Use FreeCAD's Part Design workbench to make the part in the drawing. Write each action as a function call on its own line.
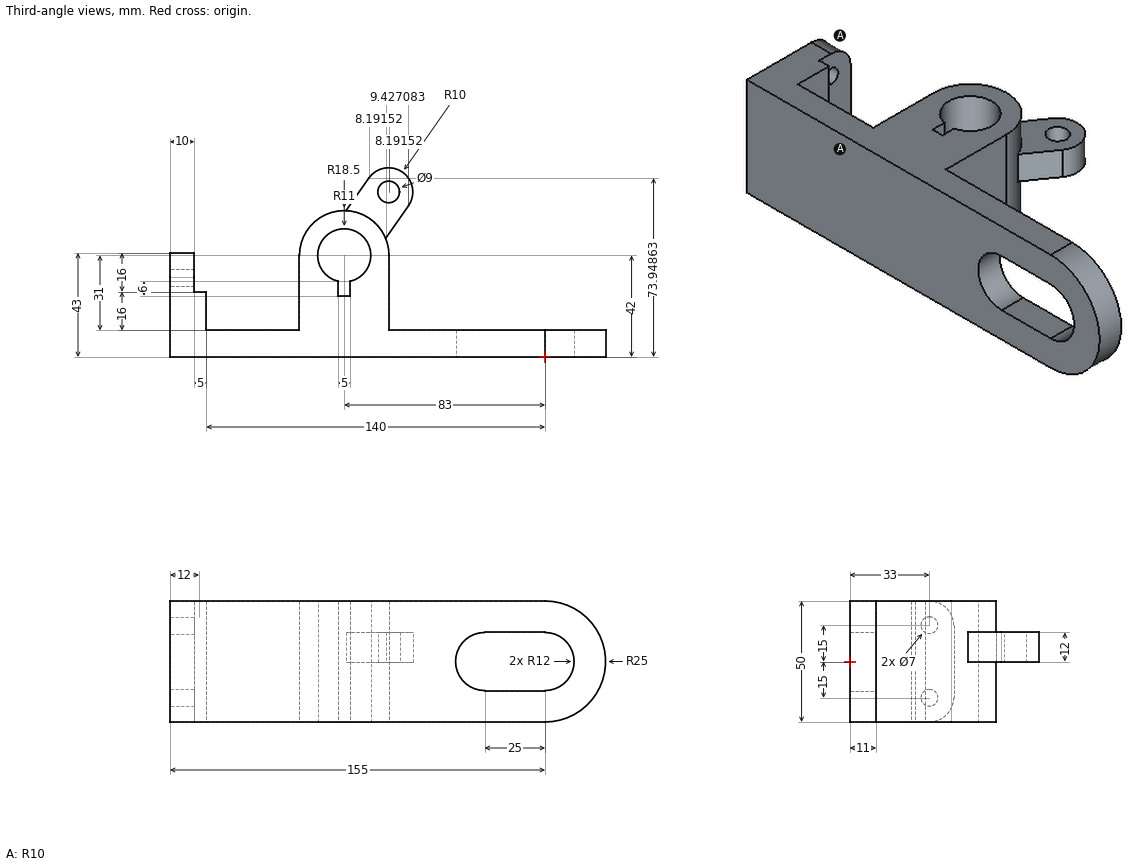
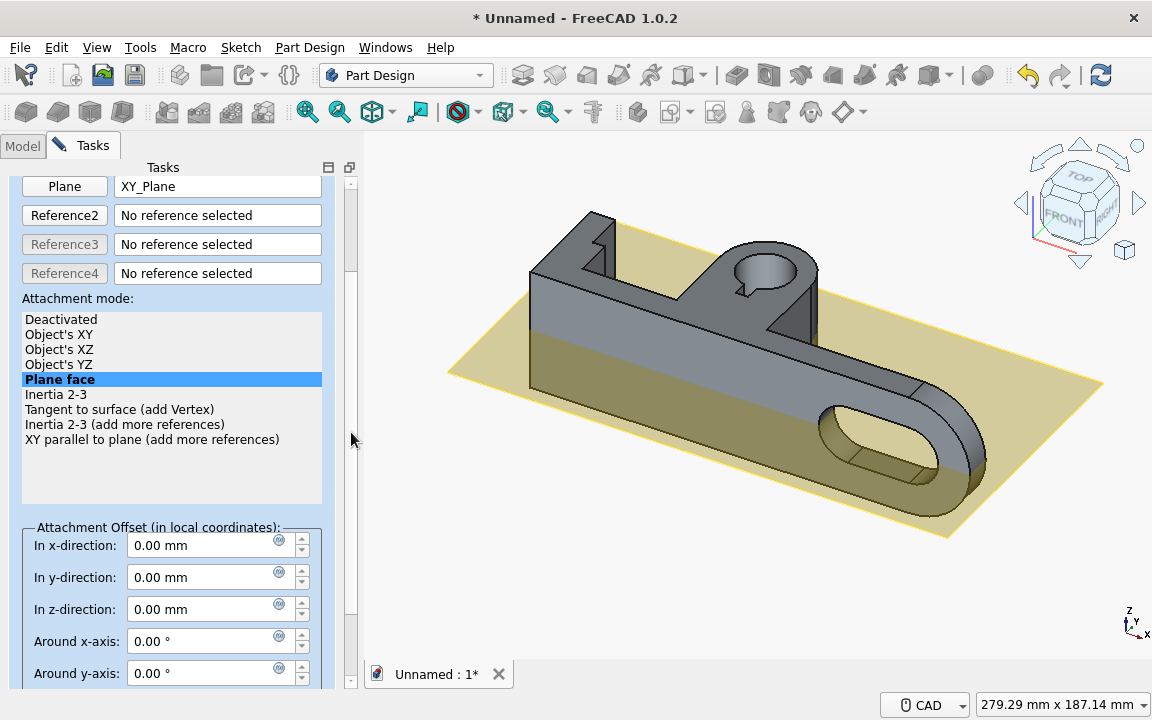
triple_click(210, 609)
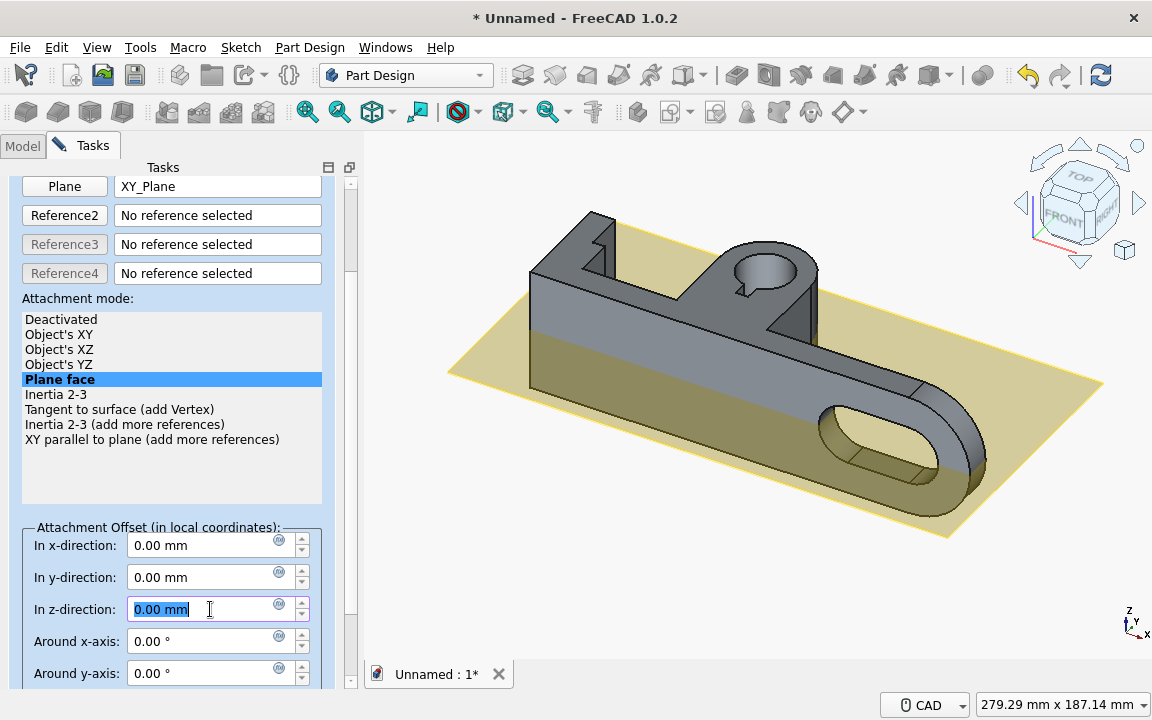
text(12)
key(Tab)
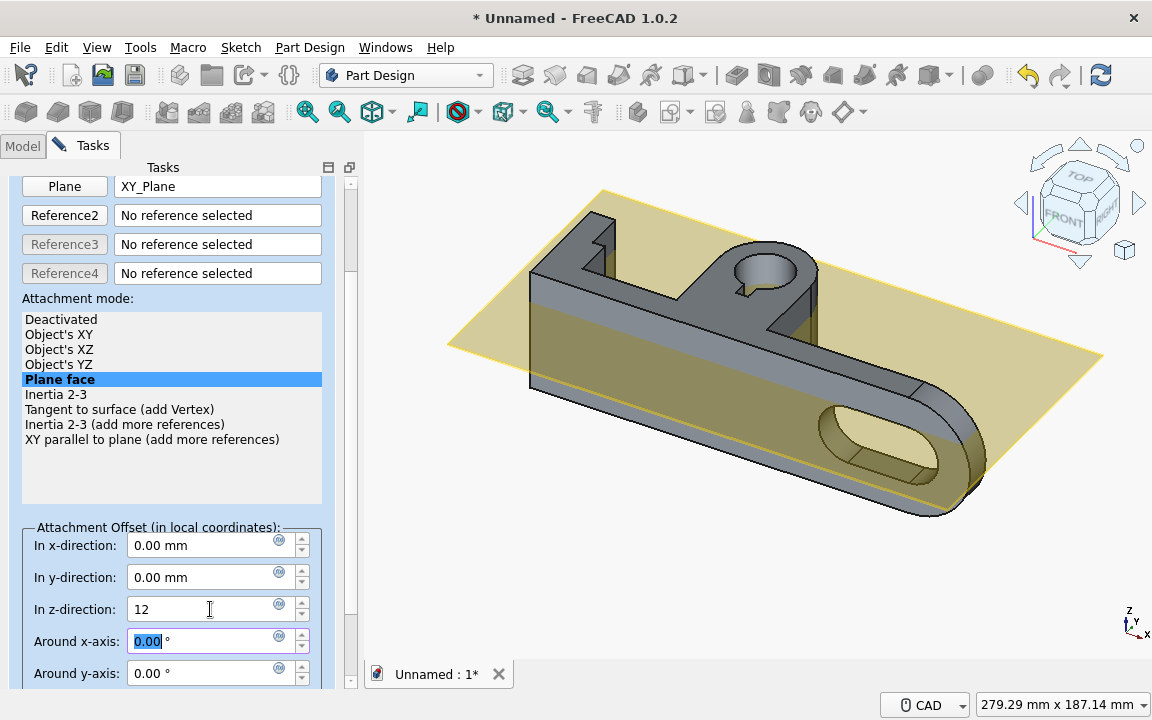
scroll(351, 432, up, 3)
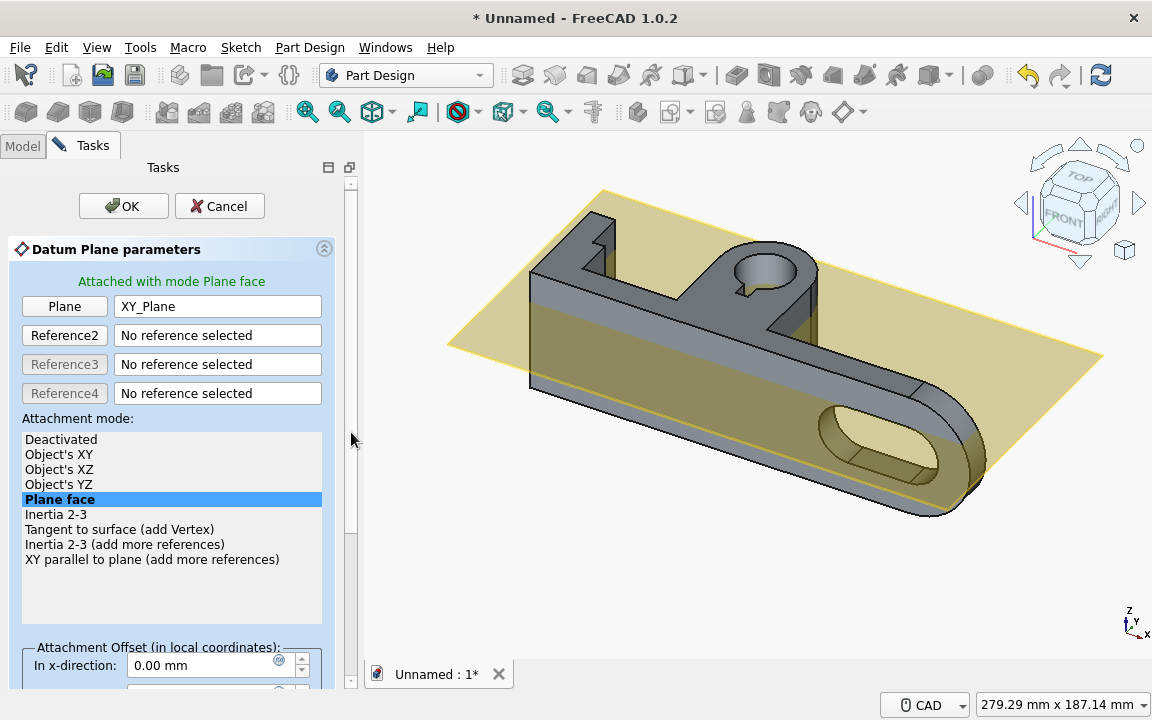
click(124, 206)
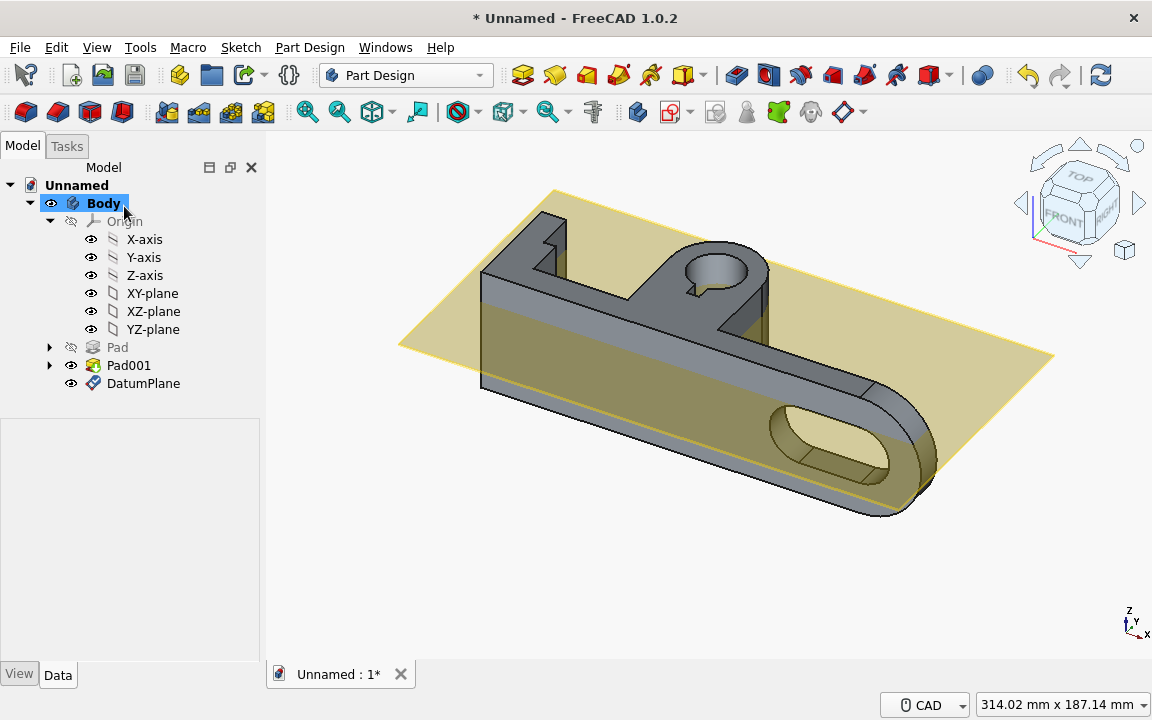
click(116, 383)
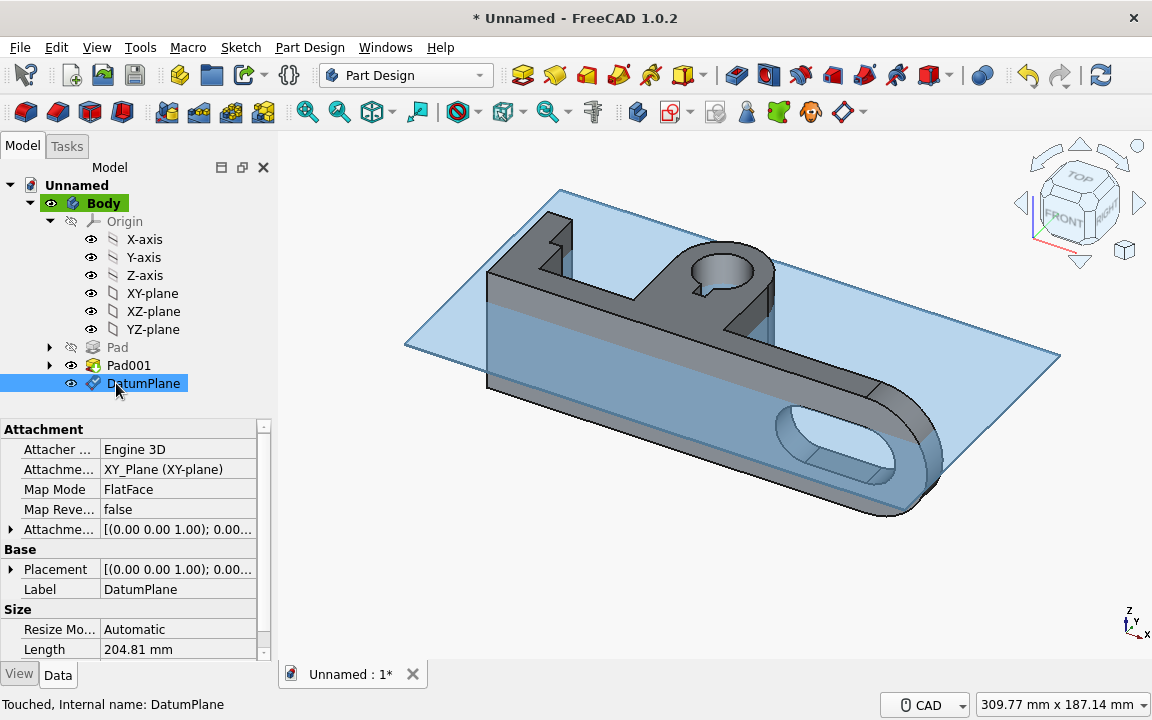
click(670, 112)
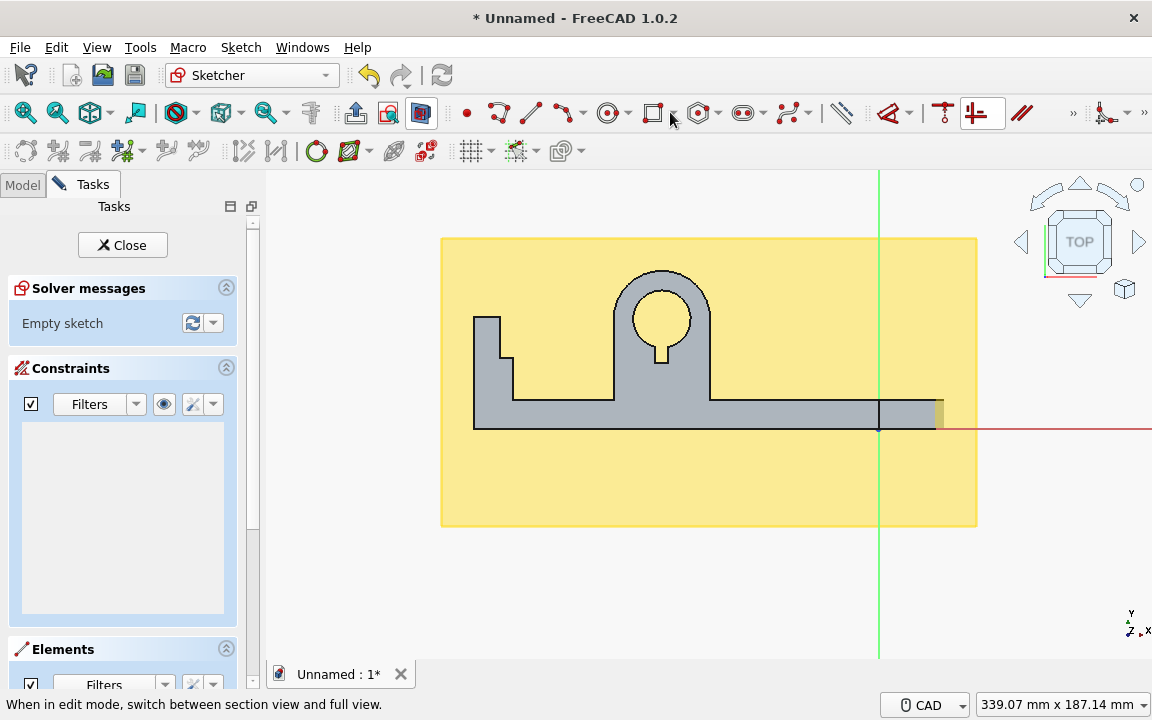
click(422, 114)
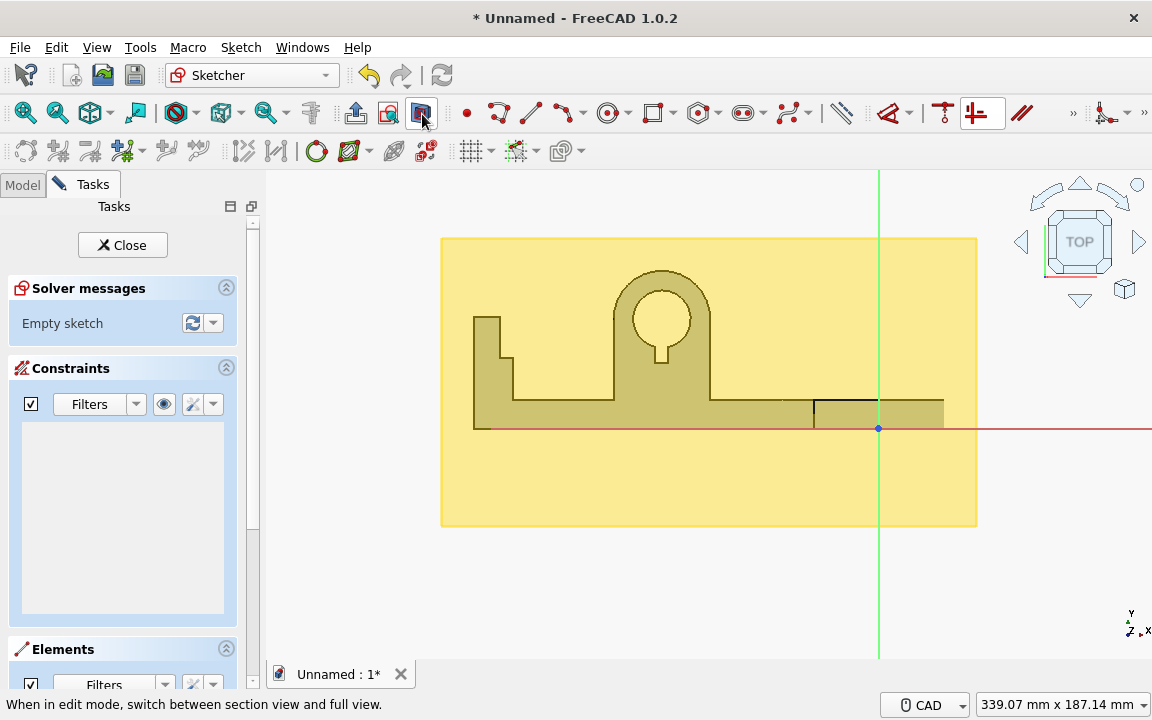
scroll(716, 216, up, 7)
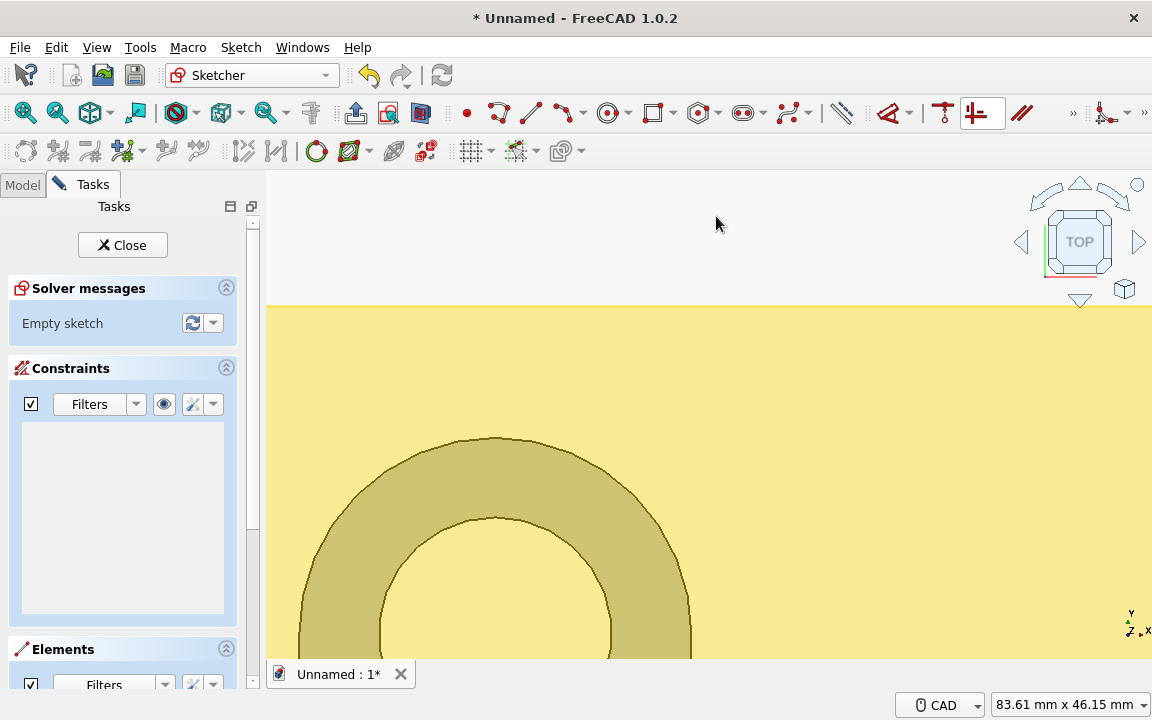
click(532, 114)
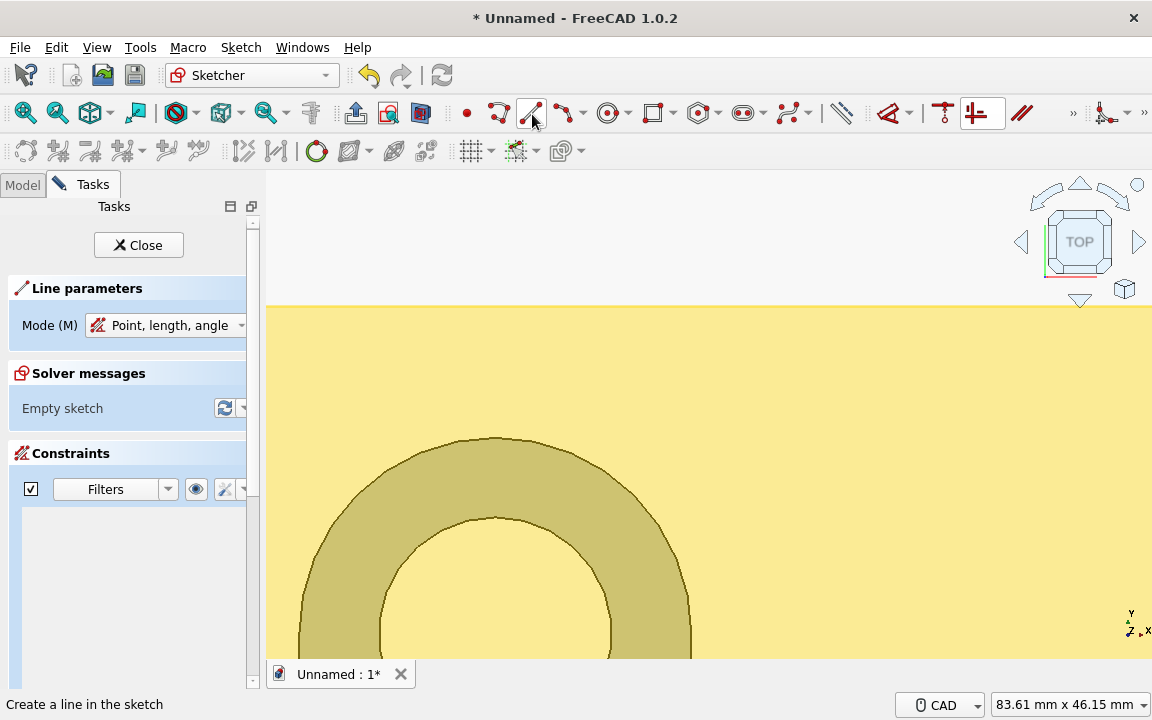
click(677, 560)
click(777, 417)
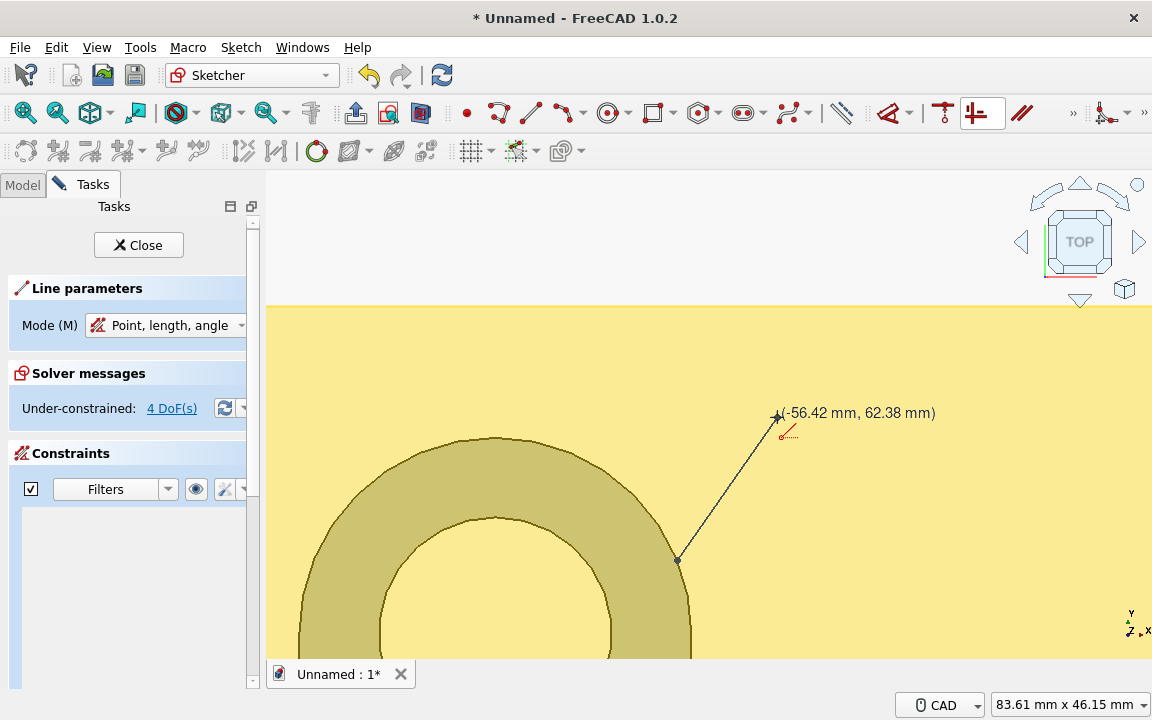
click(603, 295)
click(503, 438)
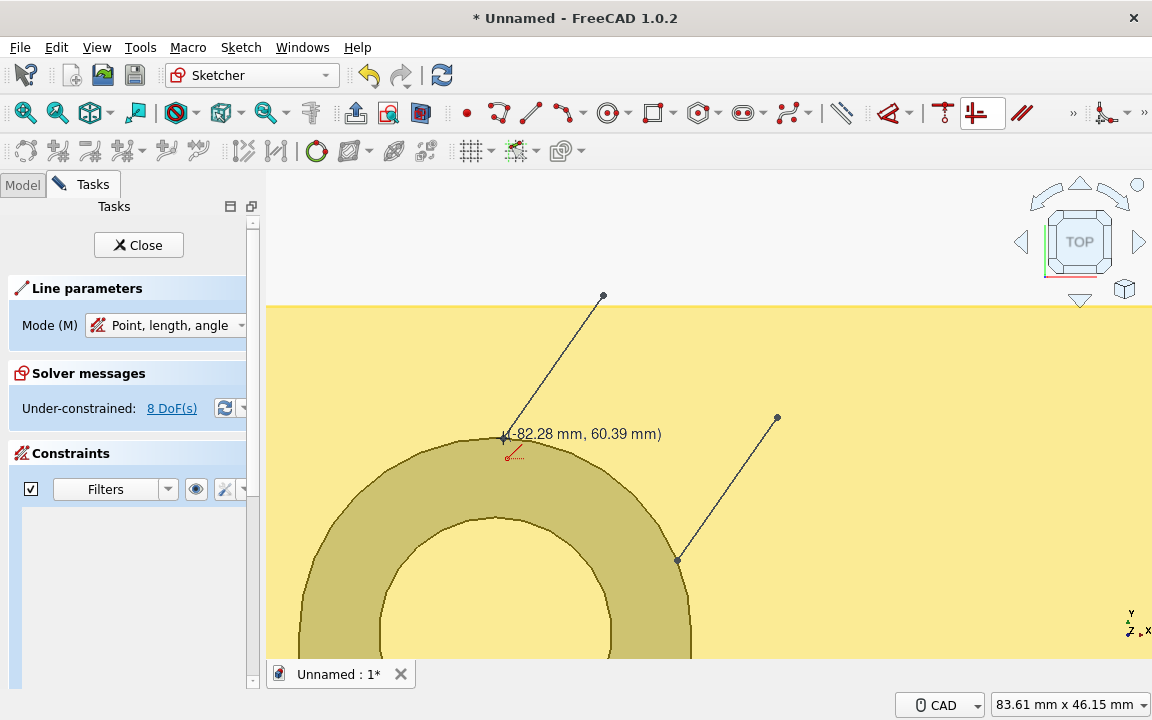
click(564, 114)